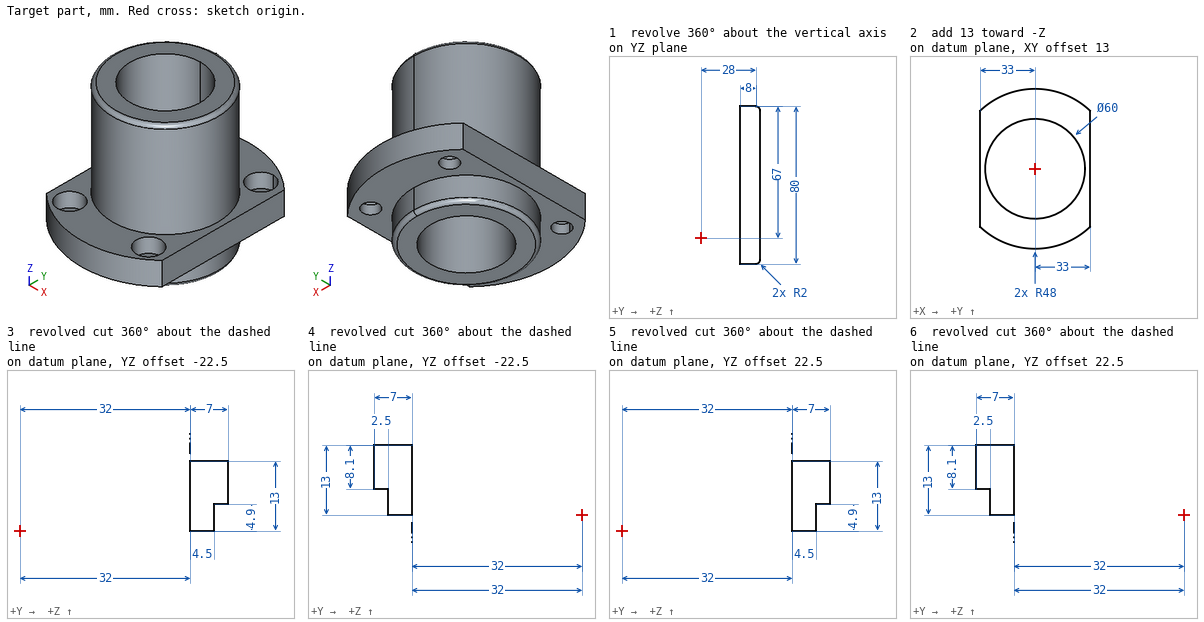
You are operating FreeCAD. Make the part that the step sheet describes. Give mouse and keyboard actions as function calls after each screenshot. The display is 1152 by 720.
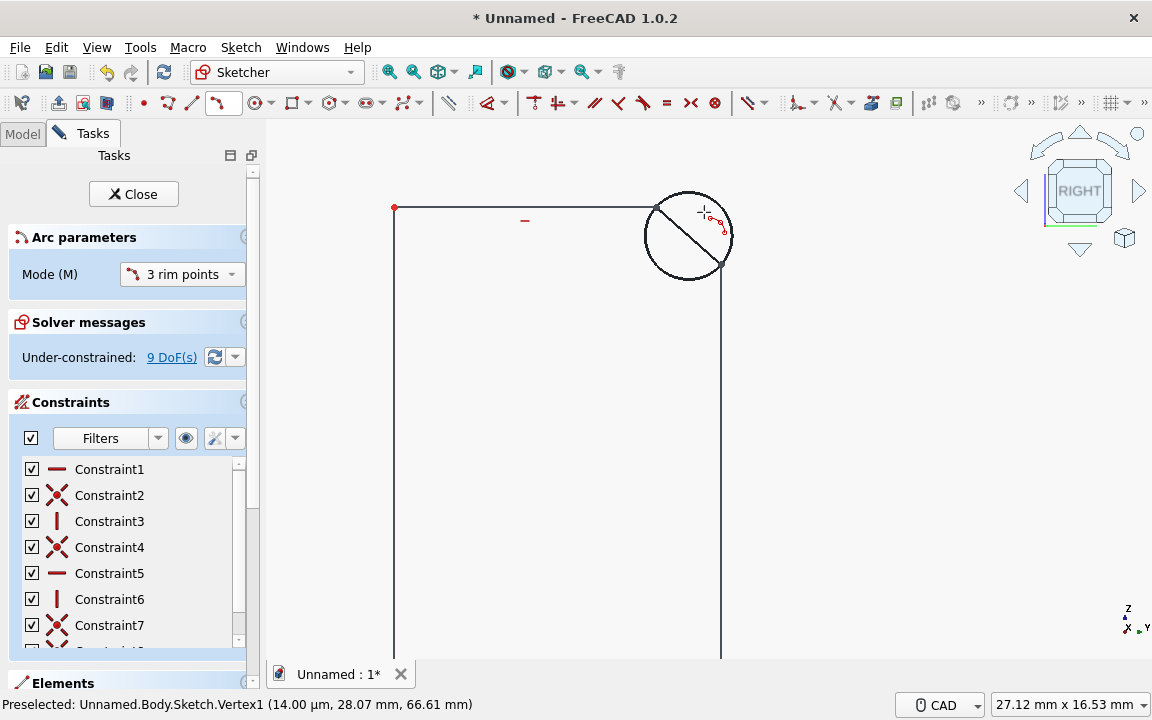
click(700, 213)
key(Escape)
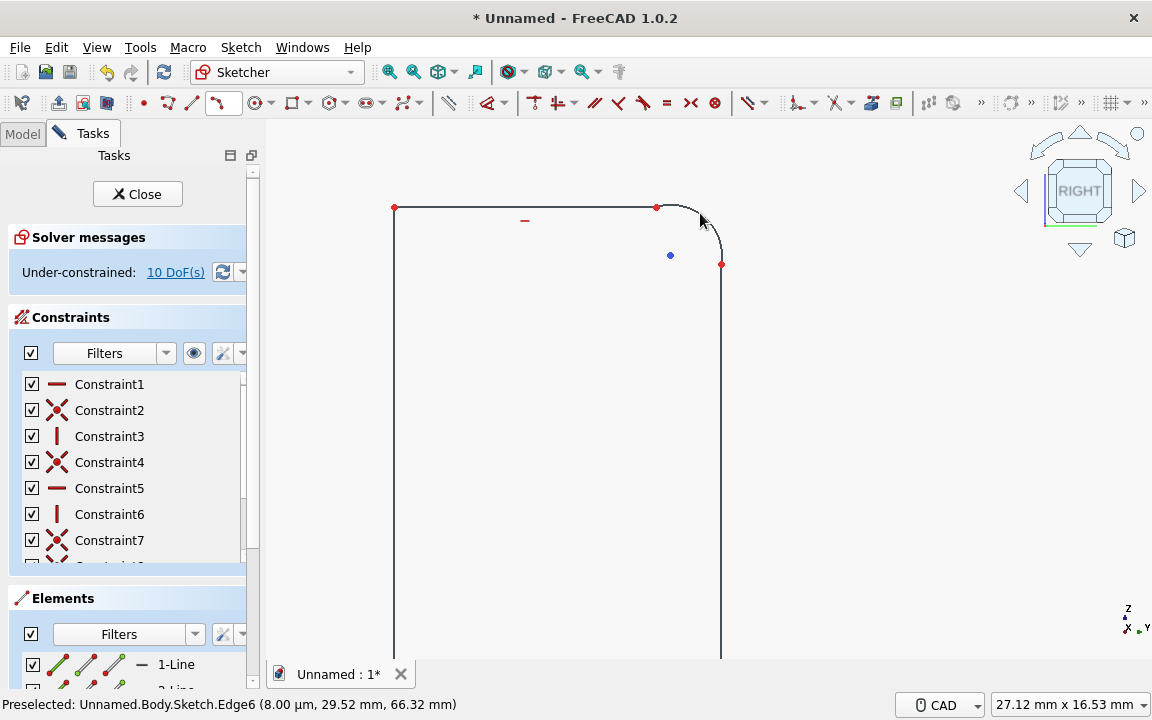
scroll(705, 215, down, 10)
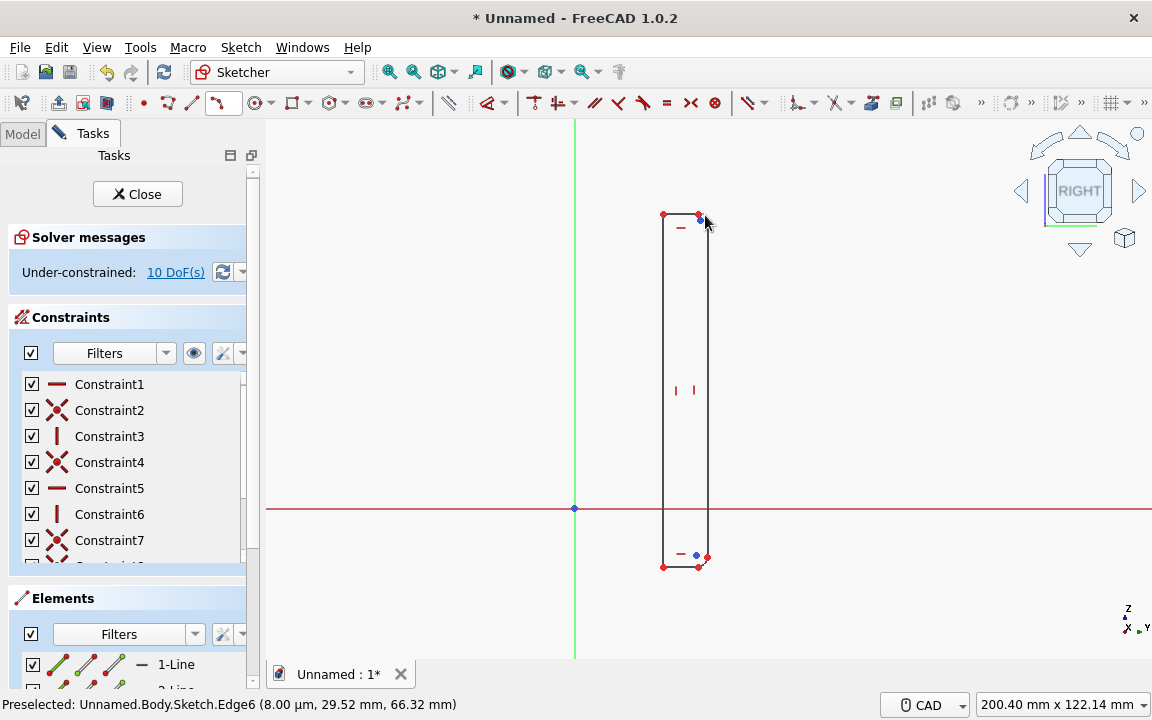
scroll(688, 214, up, 2)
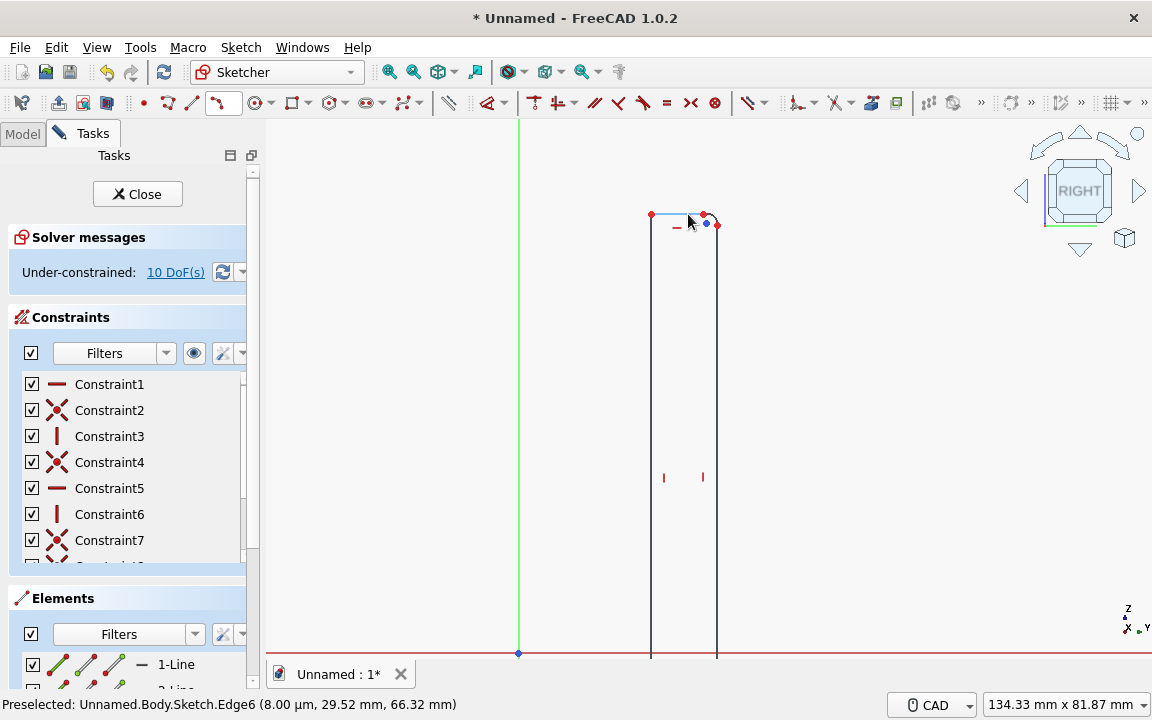
click(688, 214)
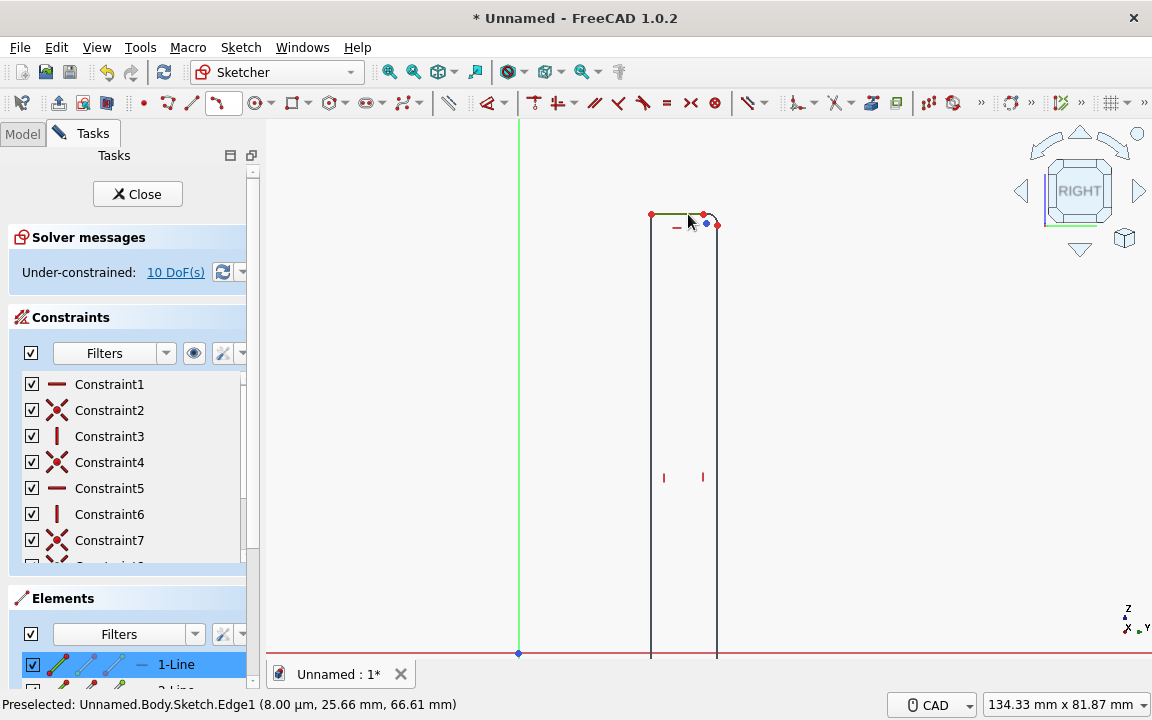
scroll(714, 216, up, 2)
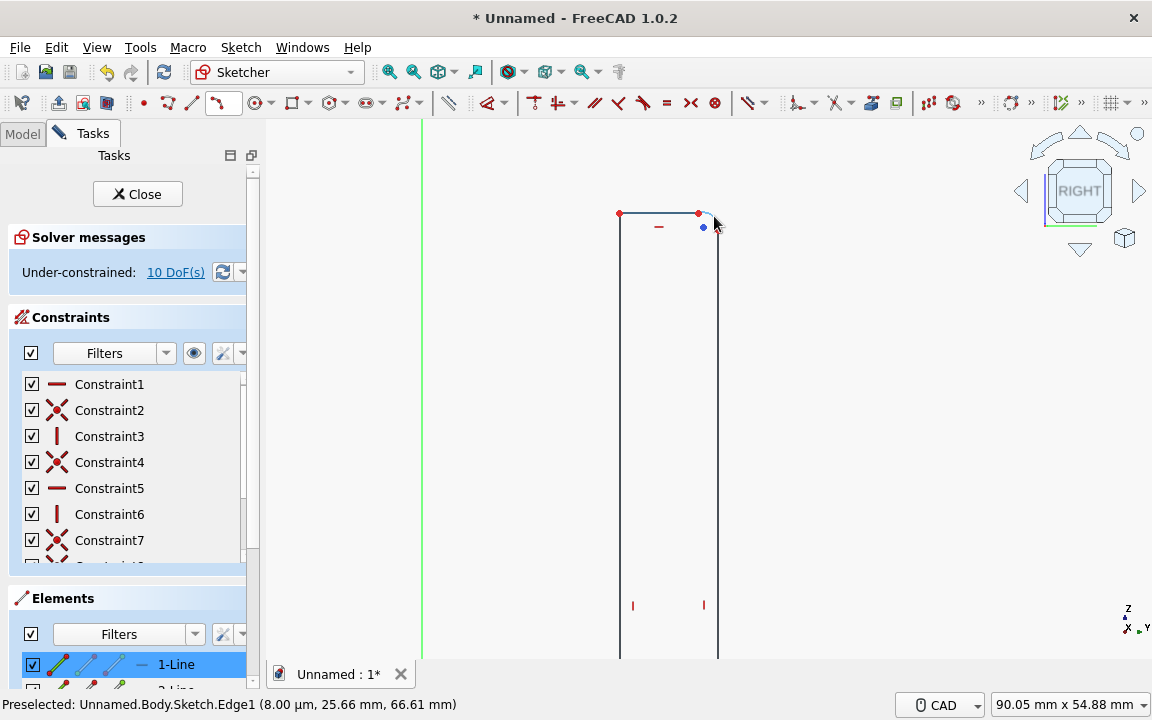
click(713, 216)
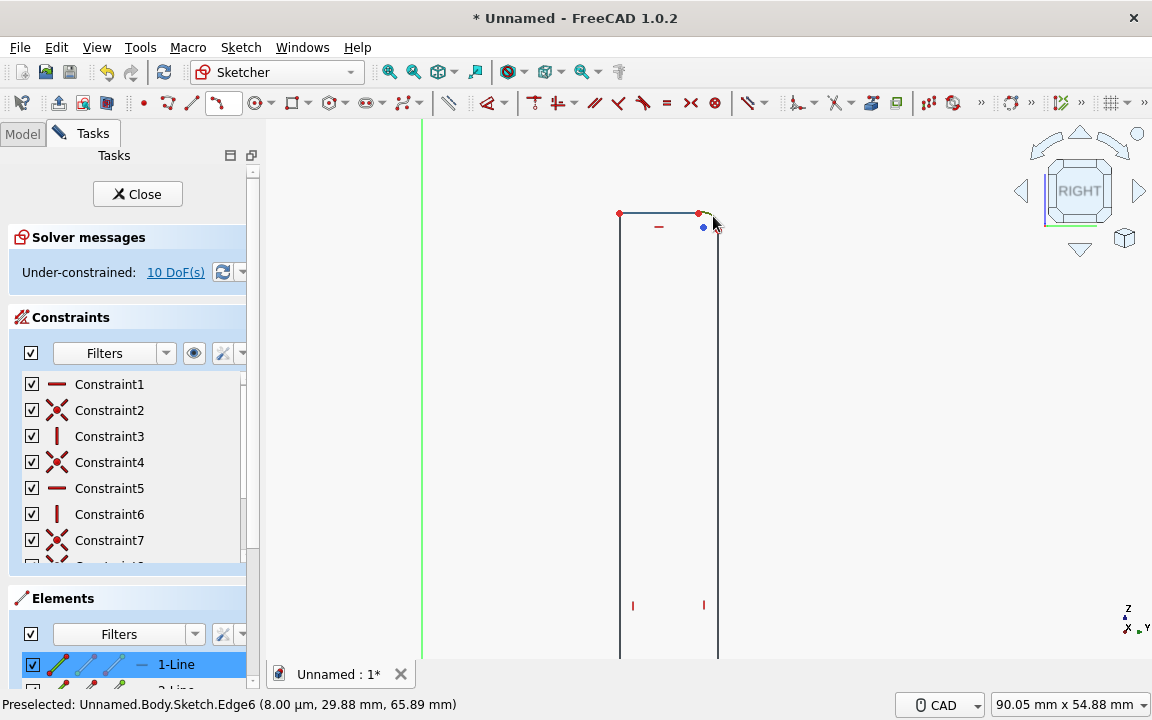
click(644, 104)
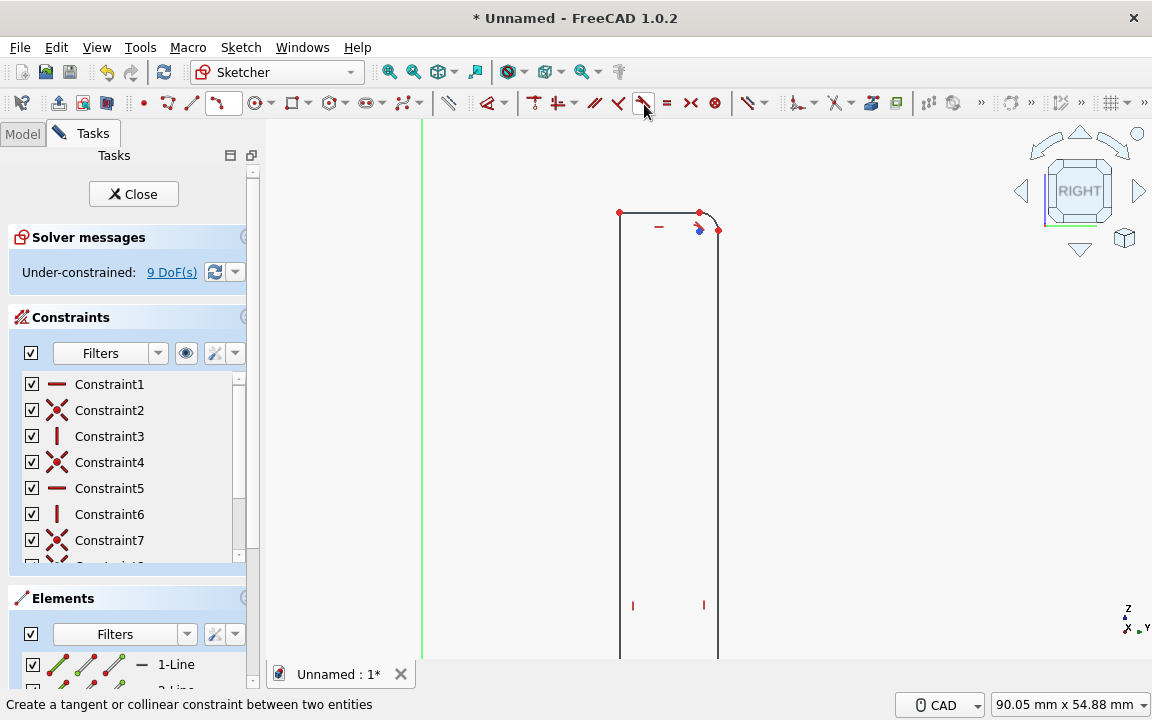
scroll(698, 215, down, 4)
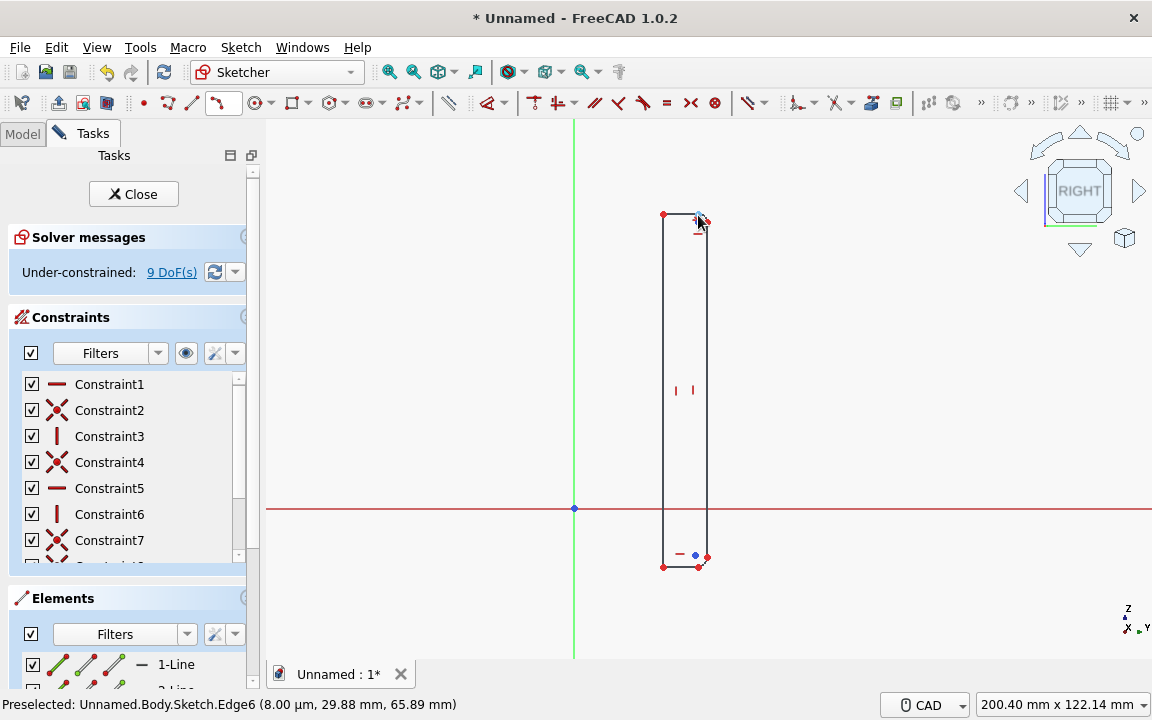
scroll(674, 567, up, 2)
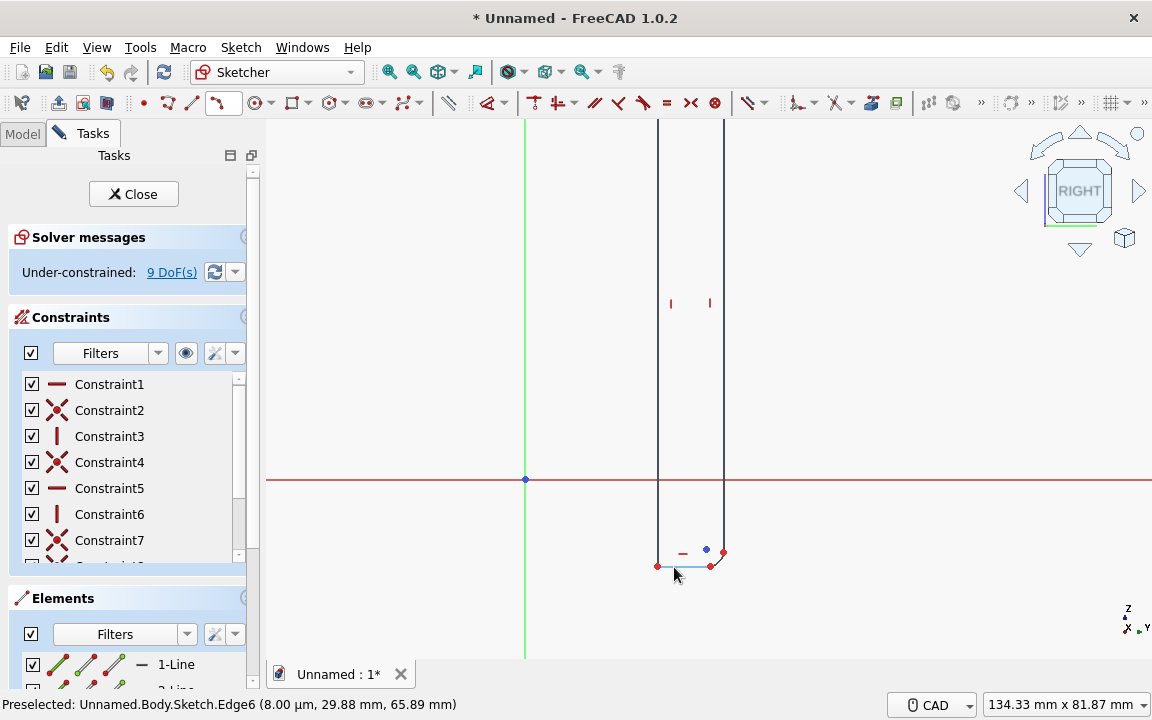
click(673, 567)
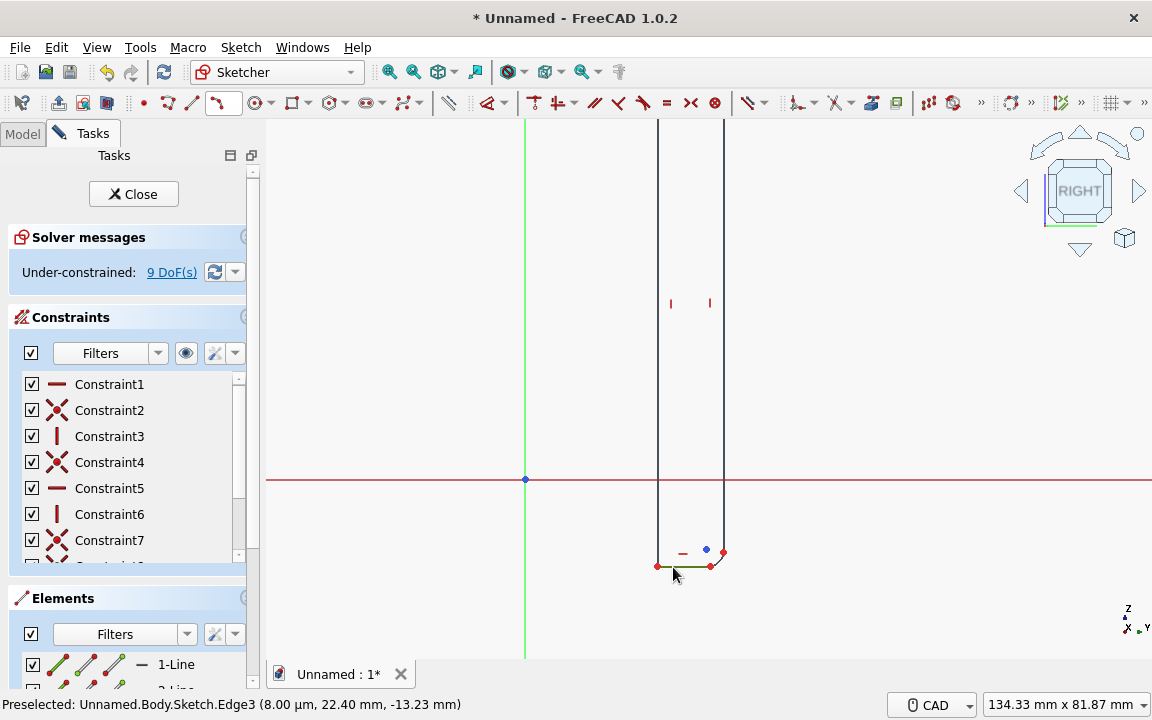
scroll(719, 562, up, 2)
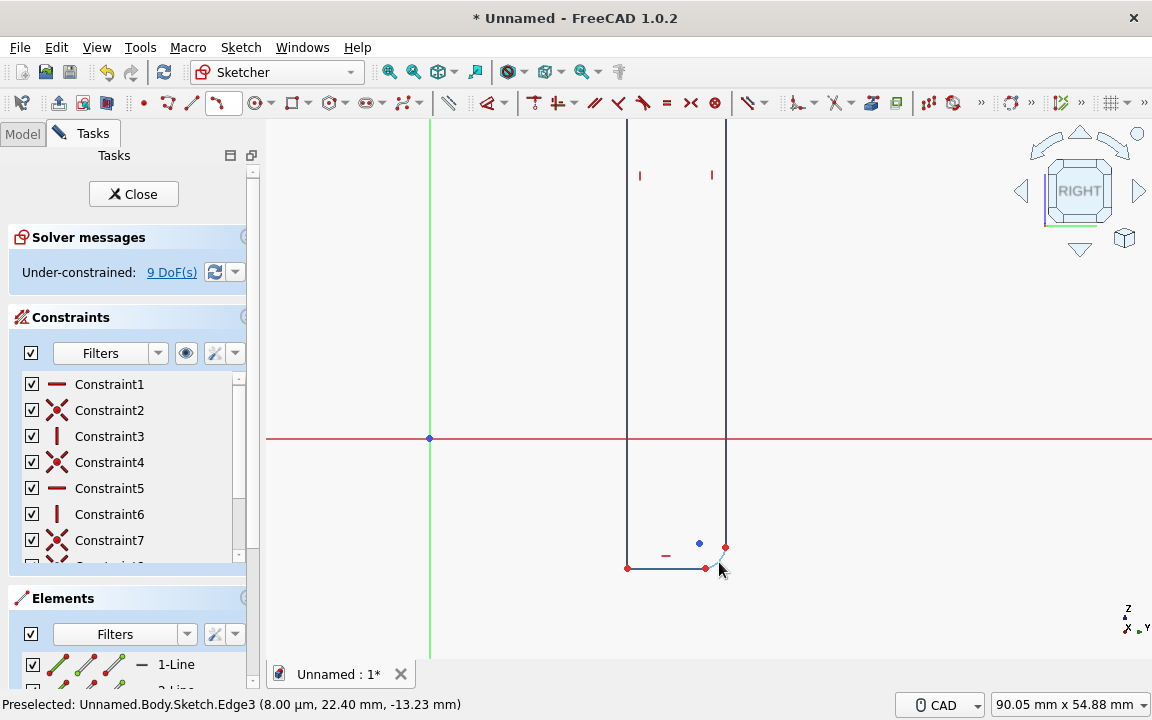
click(719, 561)